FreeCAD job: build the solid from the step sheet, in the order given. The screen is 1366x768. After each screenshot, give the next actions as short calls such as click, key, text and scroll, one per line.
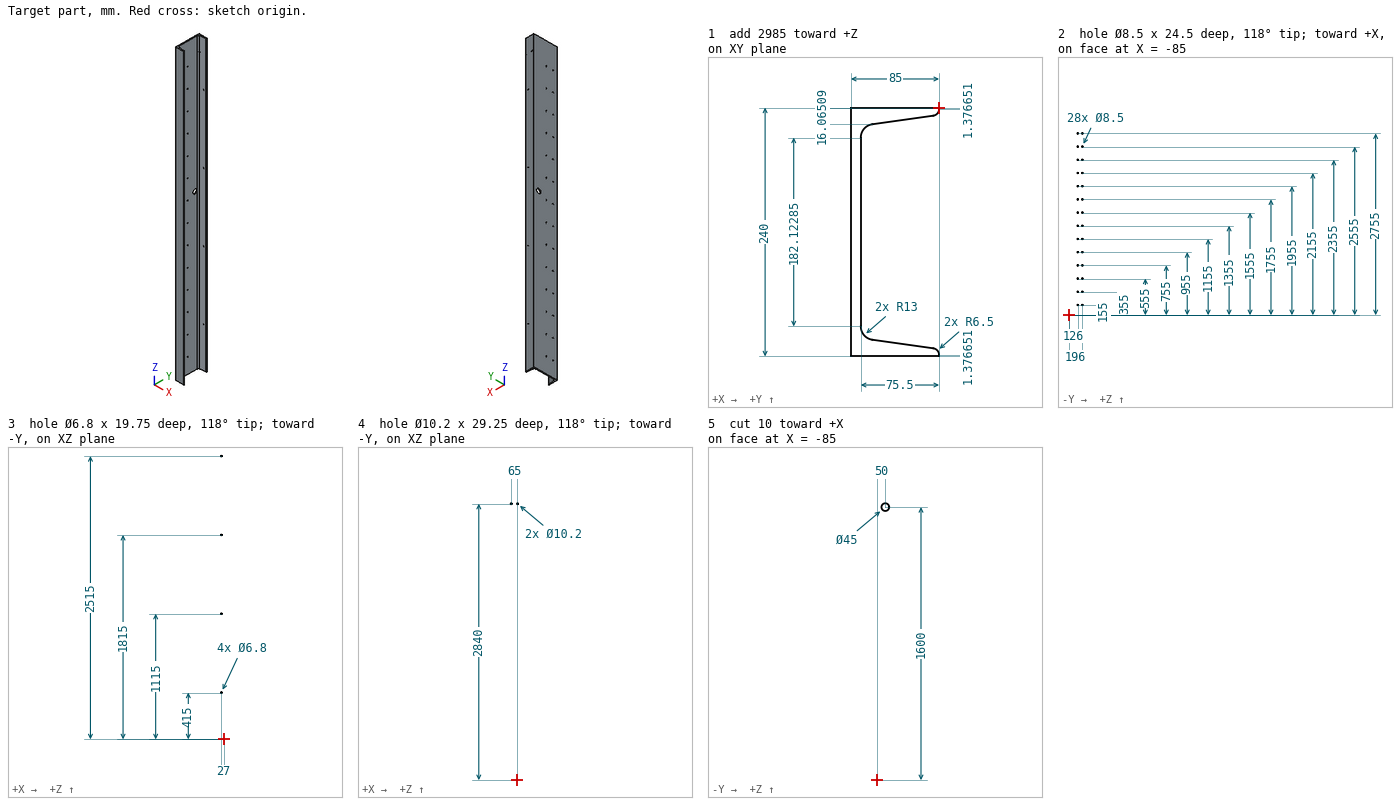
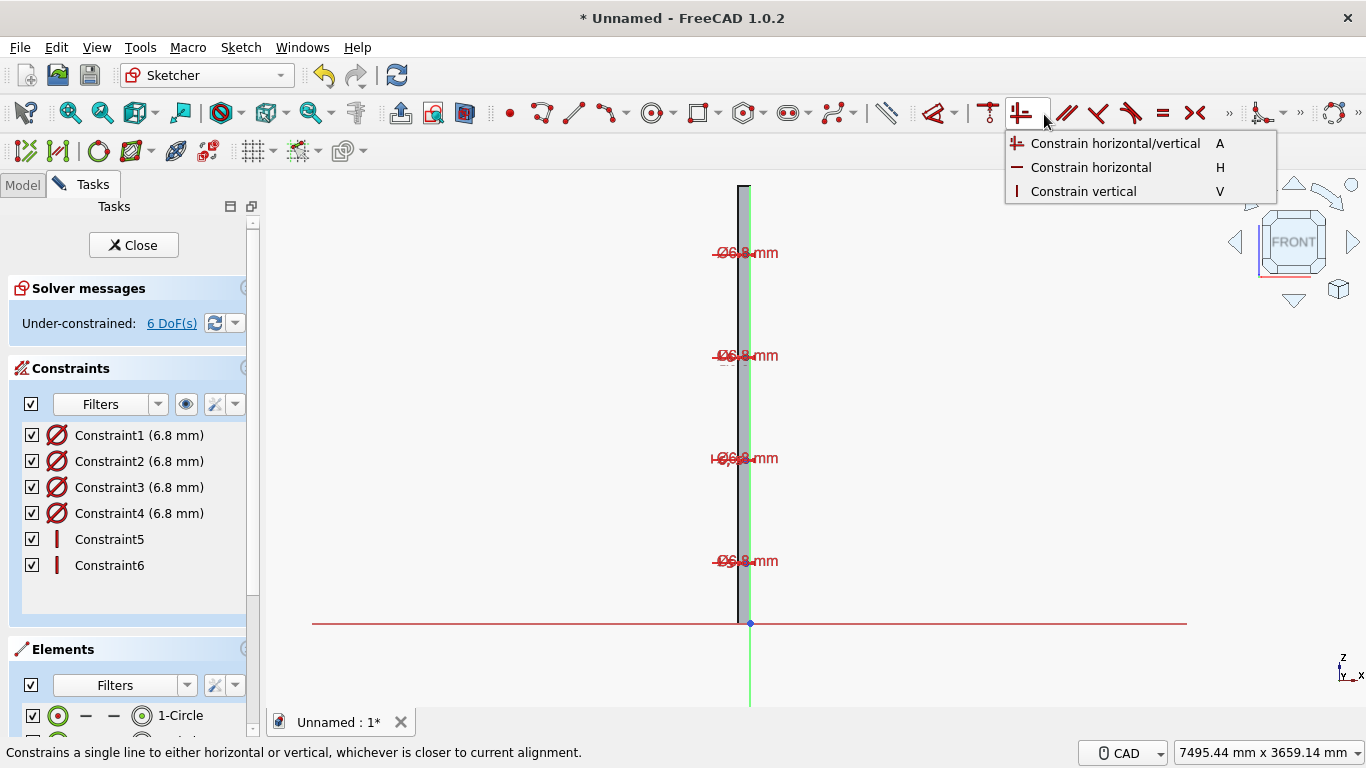
click(1141, 191)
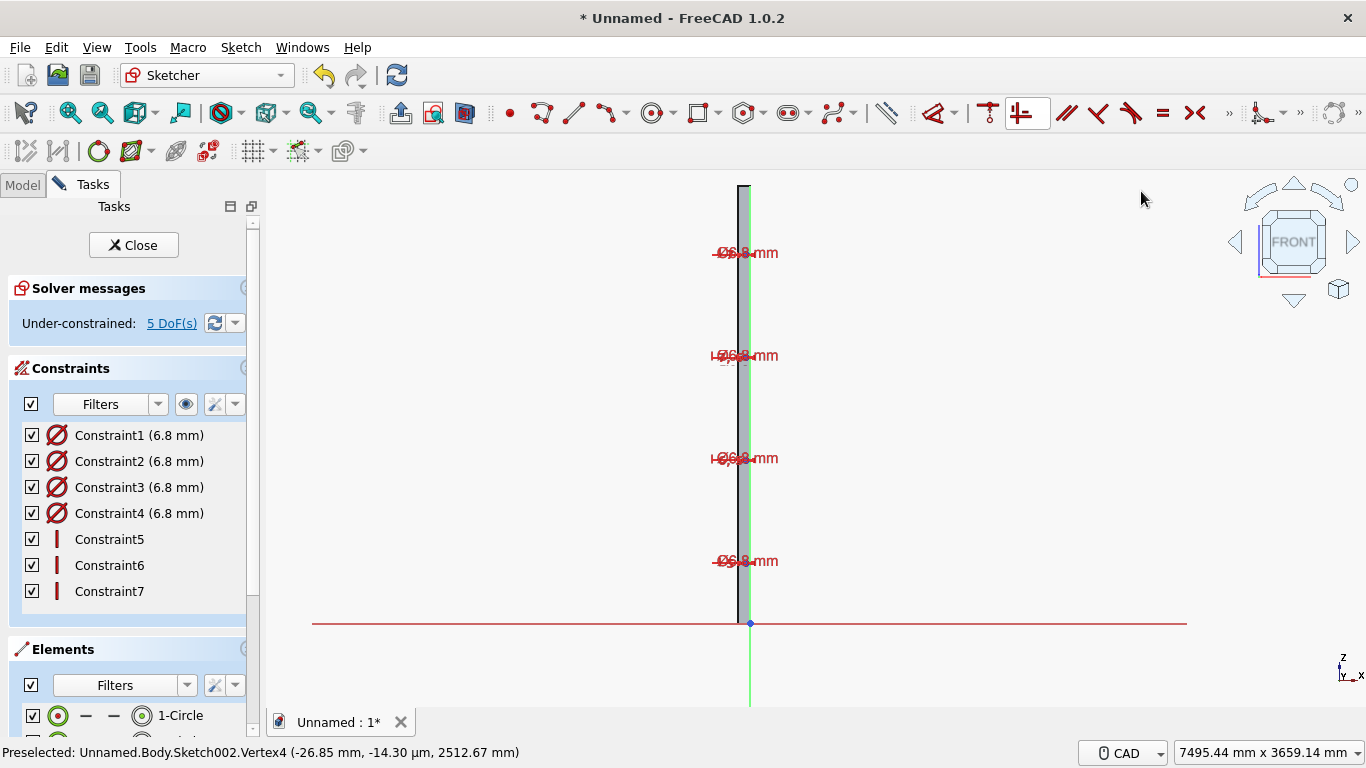
click(934, 114)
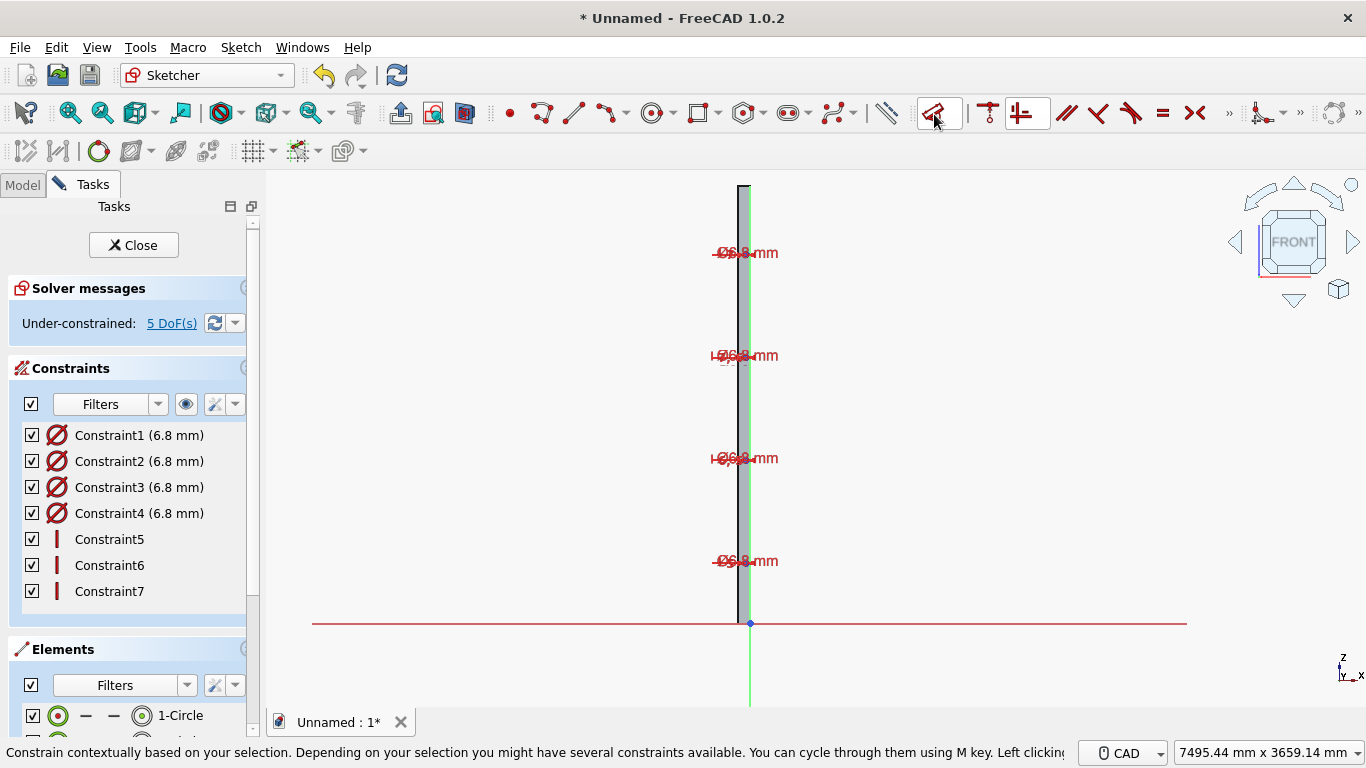
scroll(746, 563, up, 12)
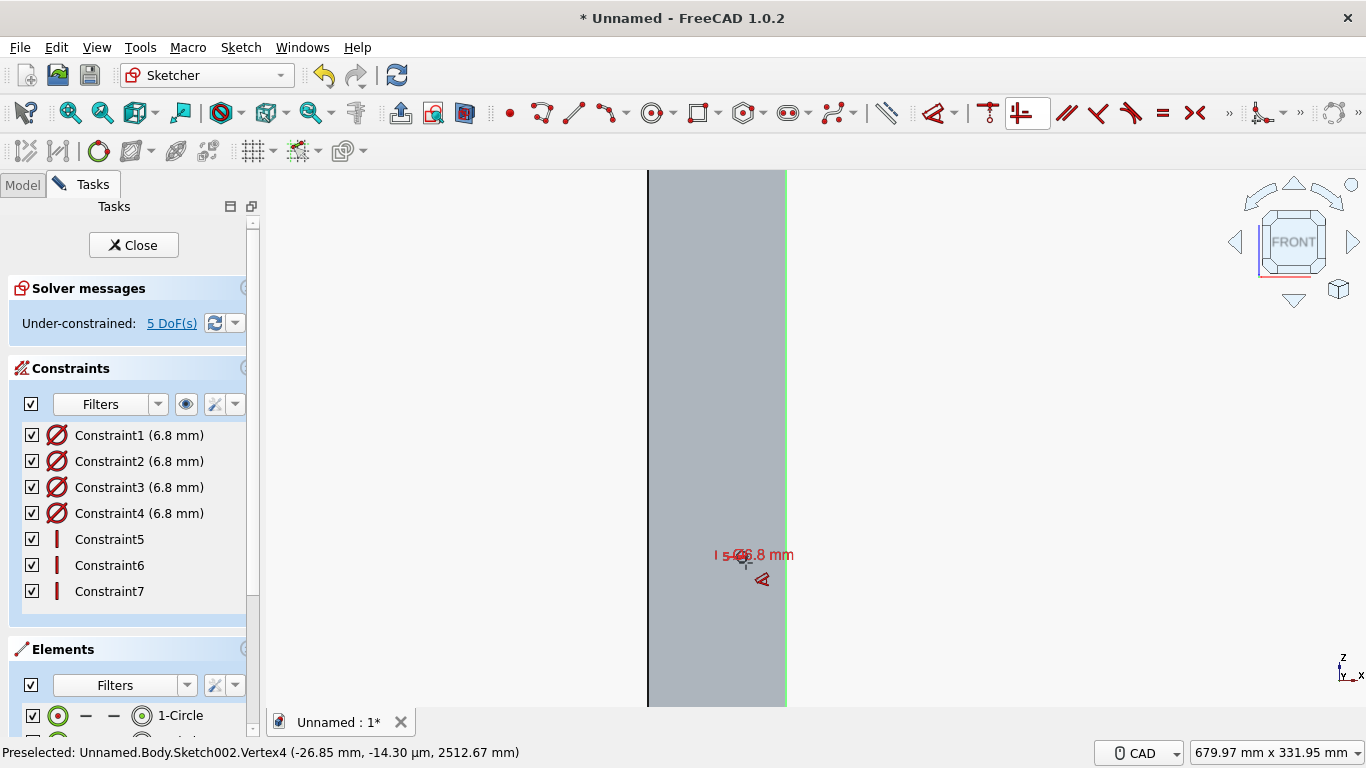
click(742, 557)
click(764, 523)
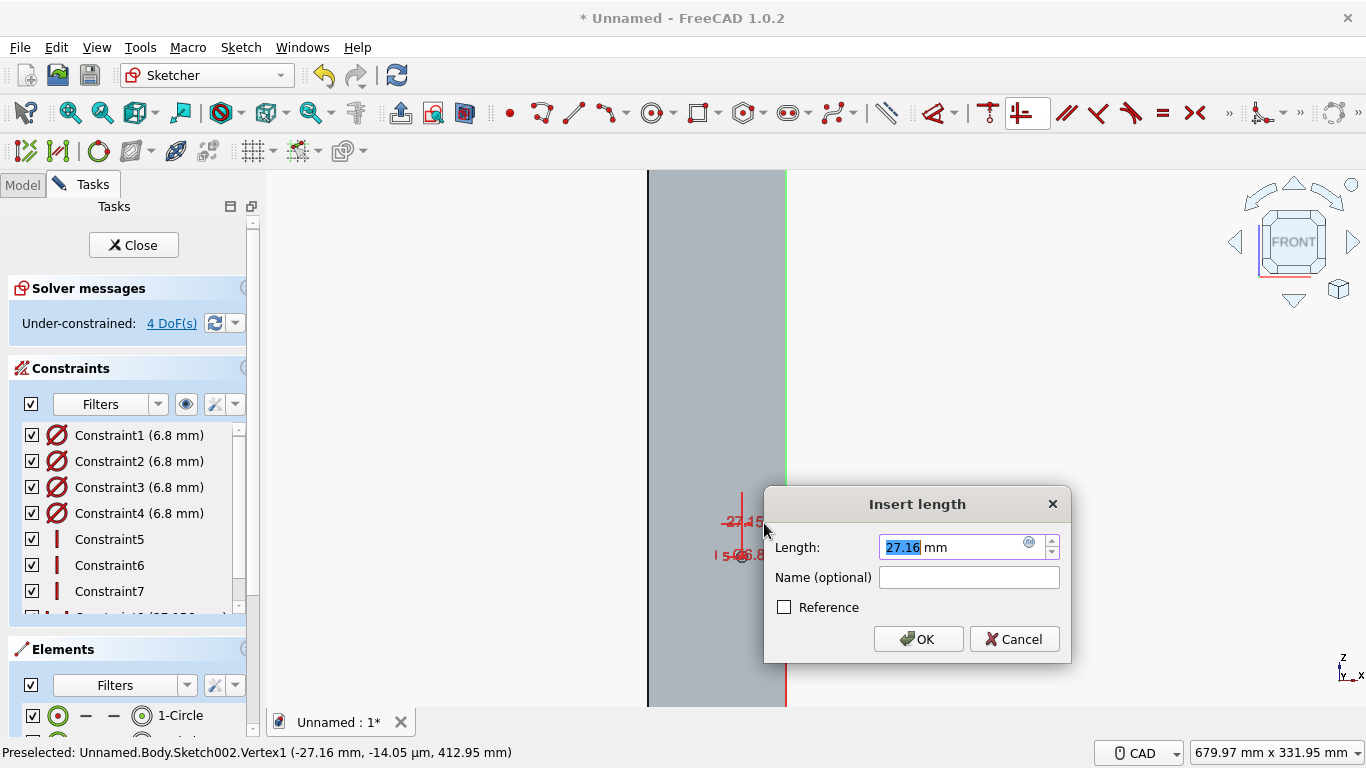
text(27)
key(Return)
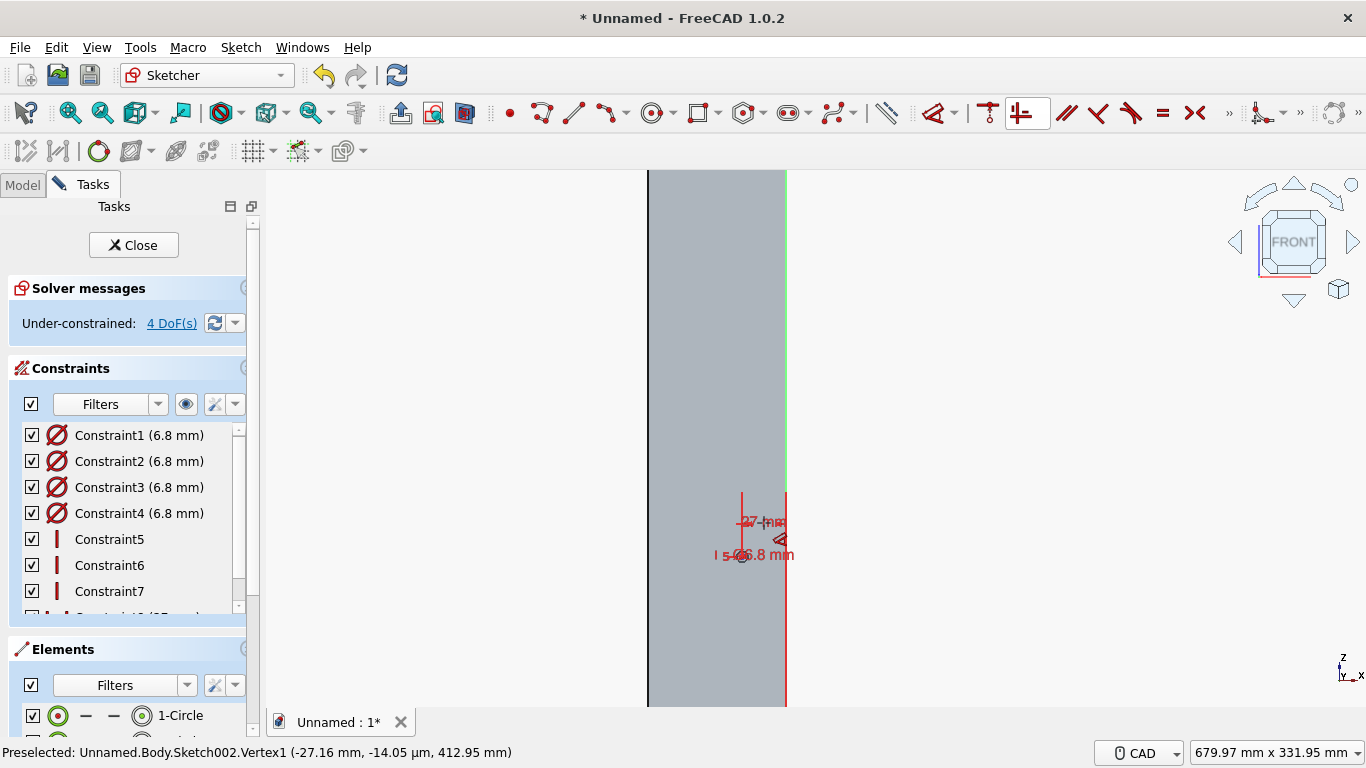
scroll(746, 563, down, 12)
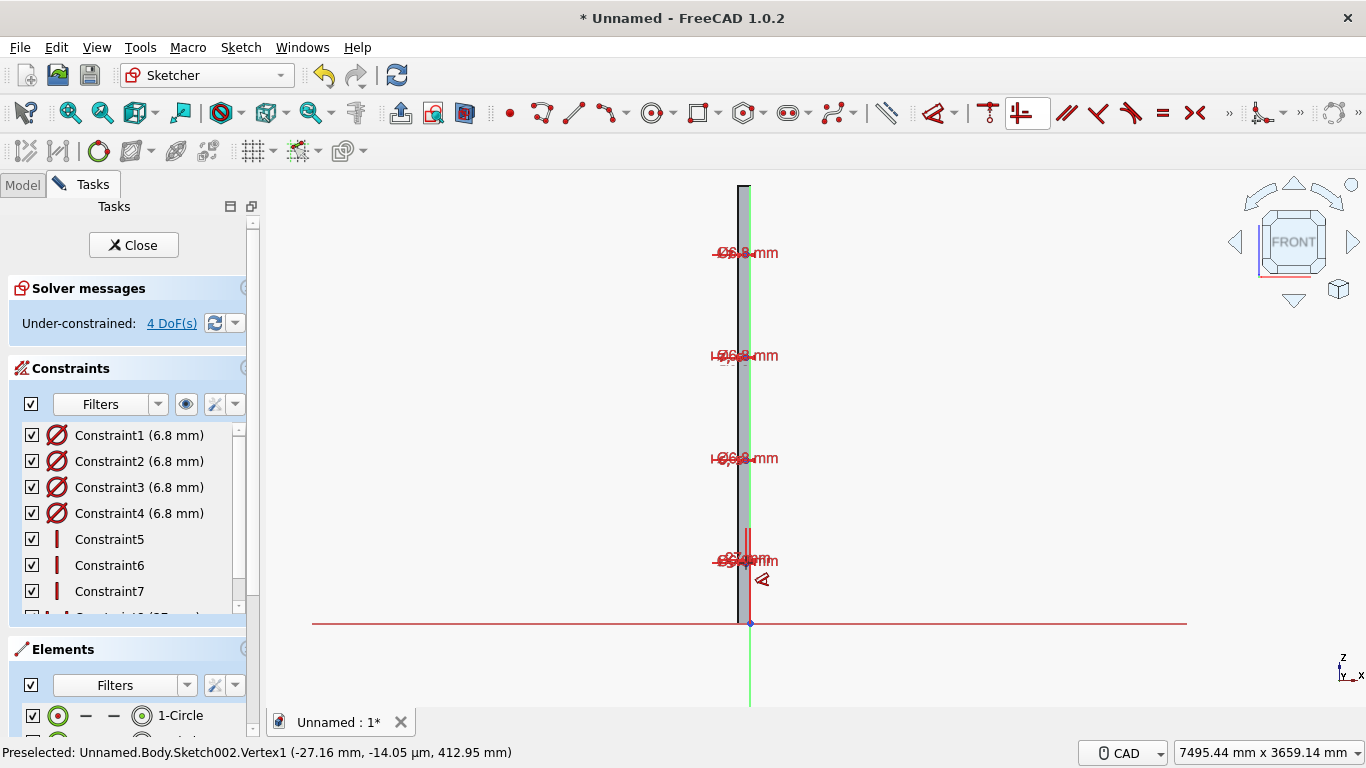
click(746, 563)
click(784, 593)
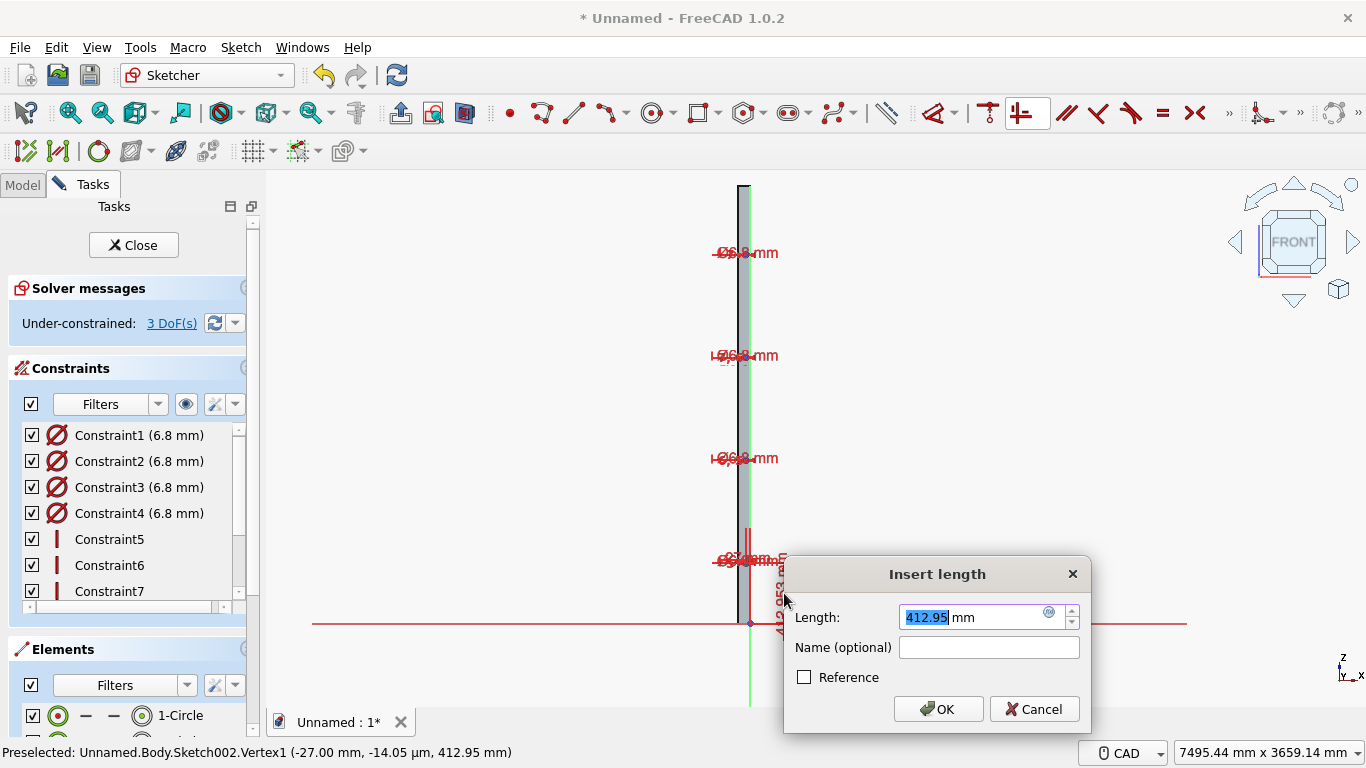
text(415)
key(Return)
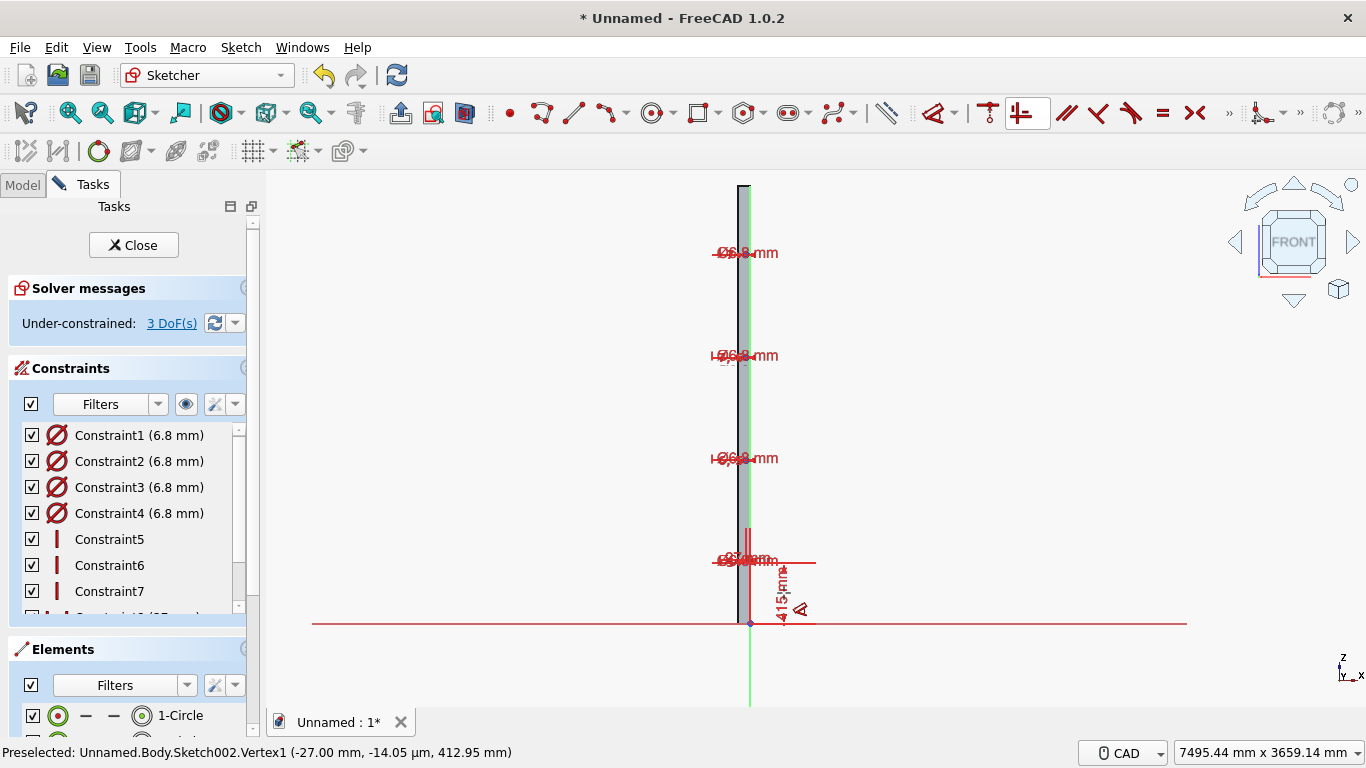
click(746, 460)
click(784, 504)